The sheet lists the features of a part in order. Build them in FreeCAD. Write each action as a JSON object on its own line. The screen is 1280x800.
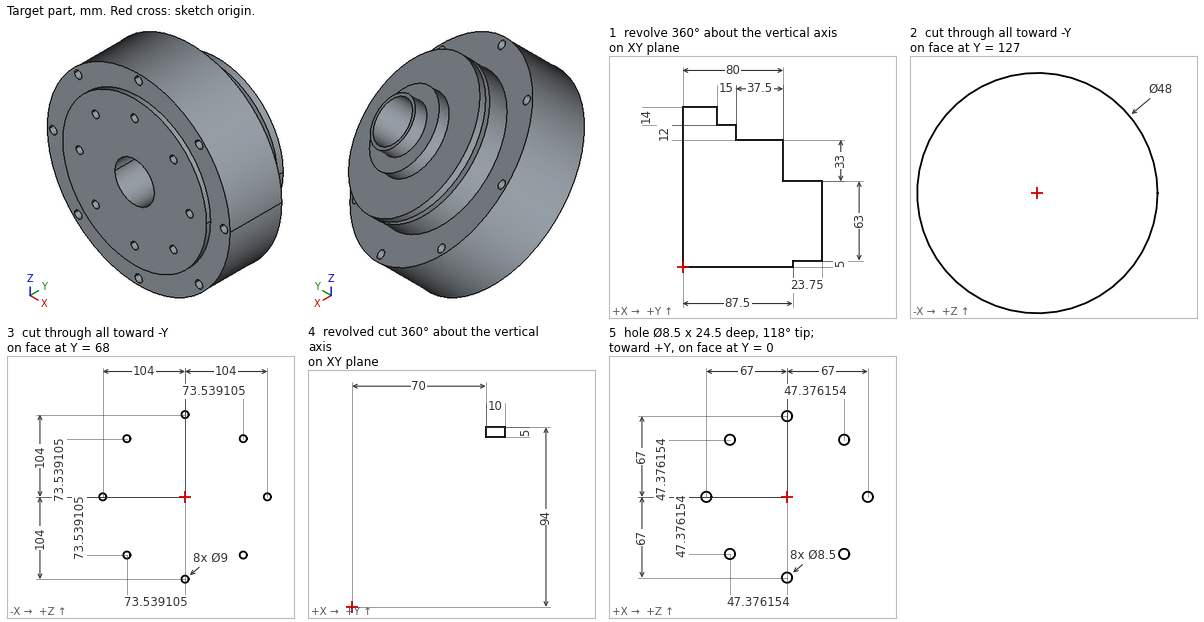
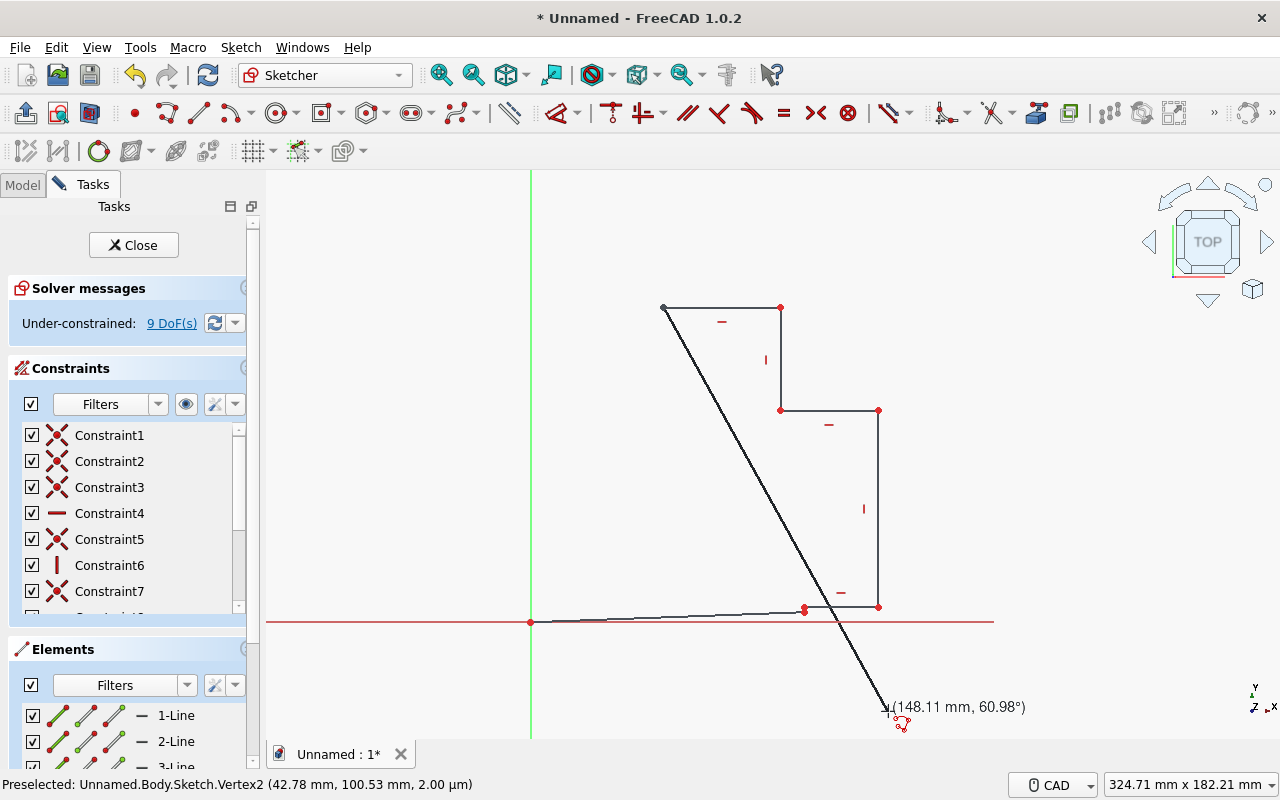
{"action": "left_click", "coordinate": [664, 269]}
{"action": "left_click", "coordinate": [617, 269]}
{"action": "left_click", "coordinate": [617, 226]}
{"action": "left_click", "coordinate": [540, 226]}
{"action": "left_click", "coordinate": [531, 622]}
{"action": "key", "text": "Escape"}
{"action": "key", "text": "Escape"}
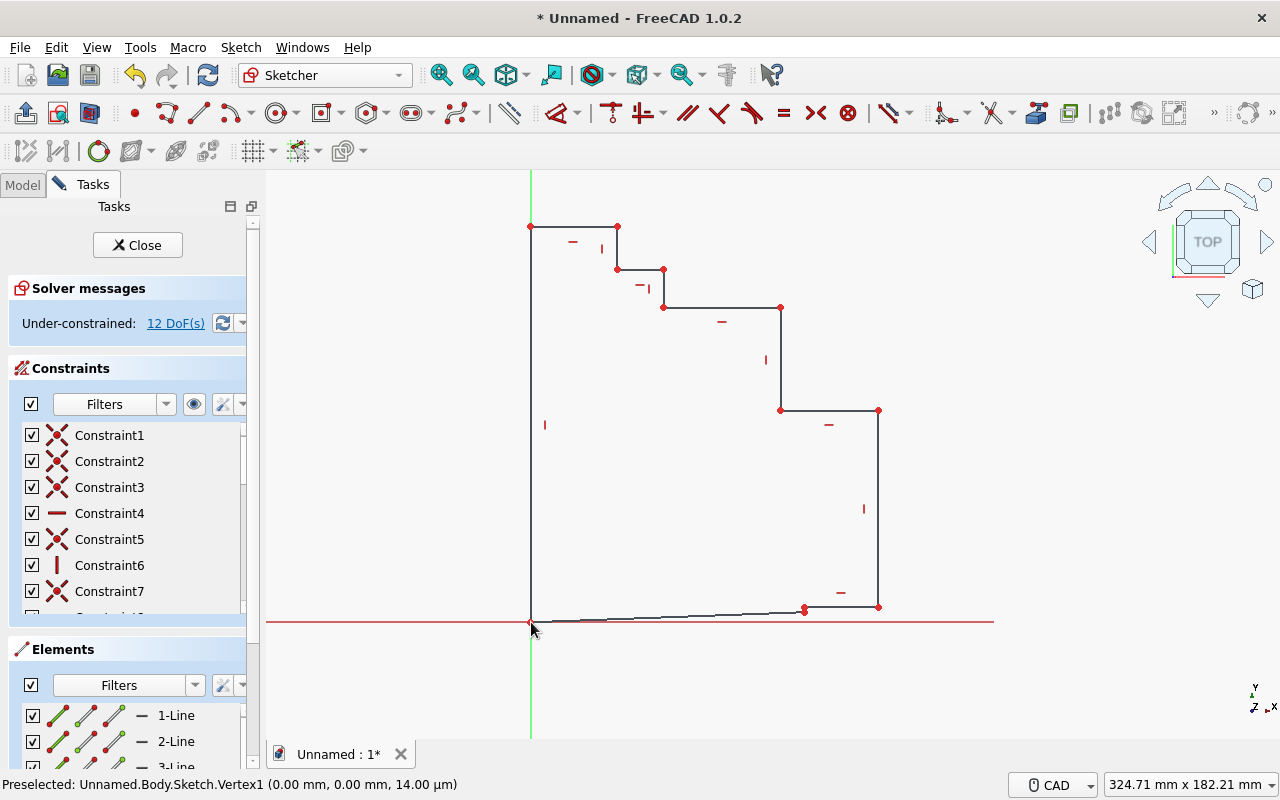
{"action": "left_click", "coordinate": [613, 619]}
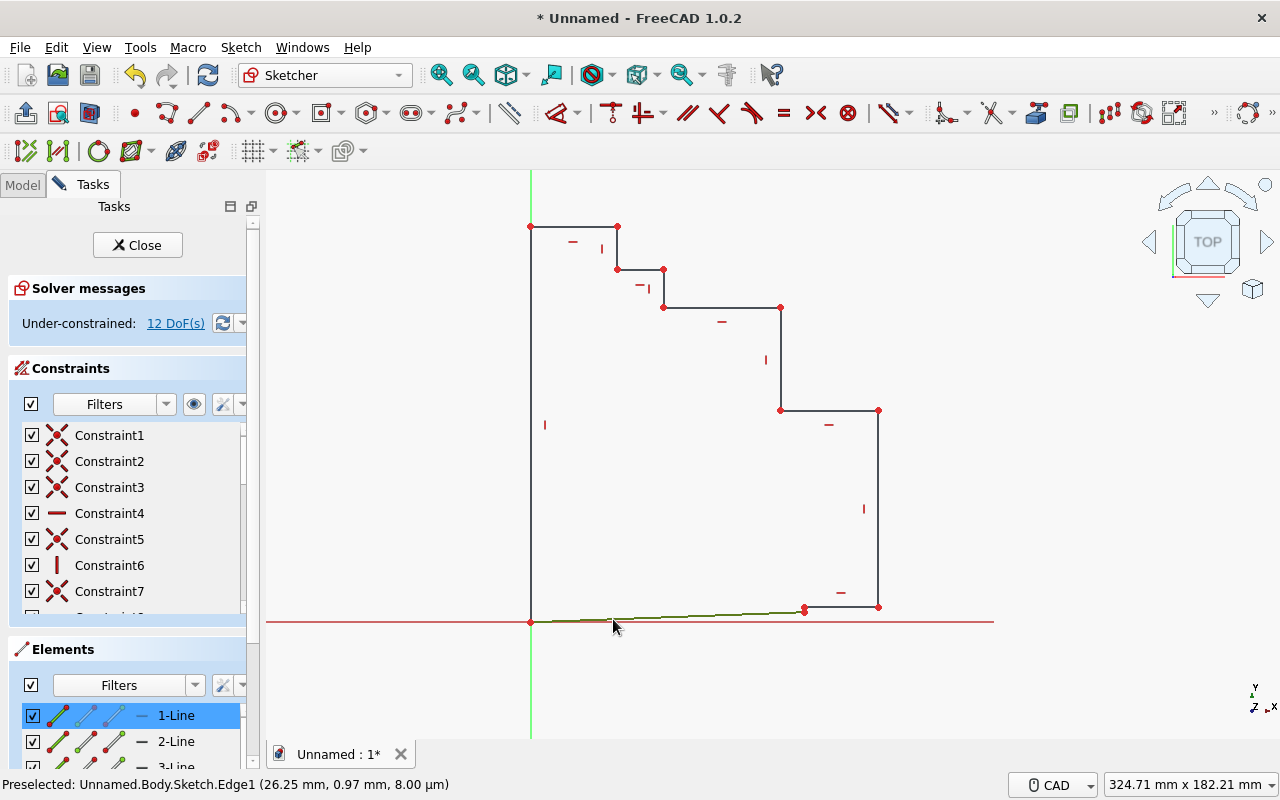
{"action": "key", "text": "h"}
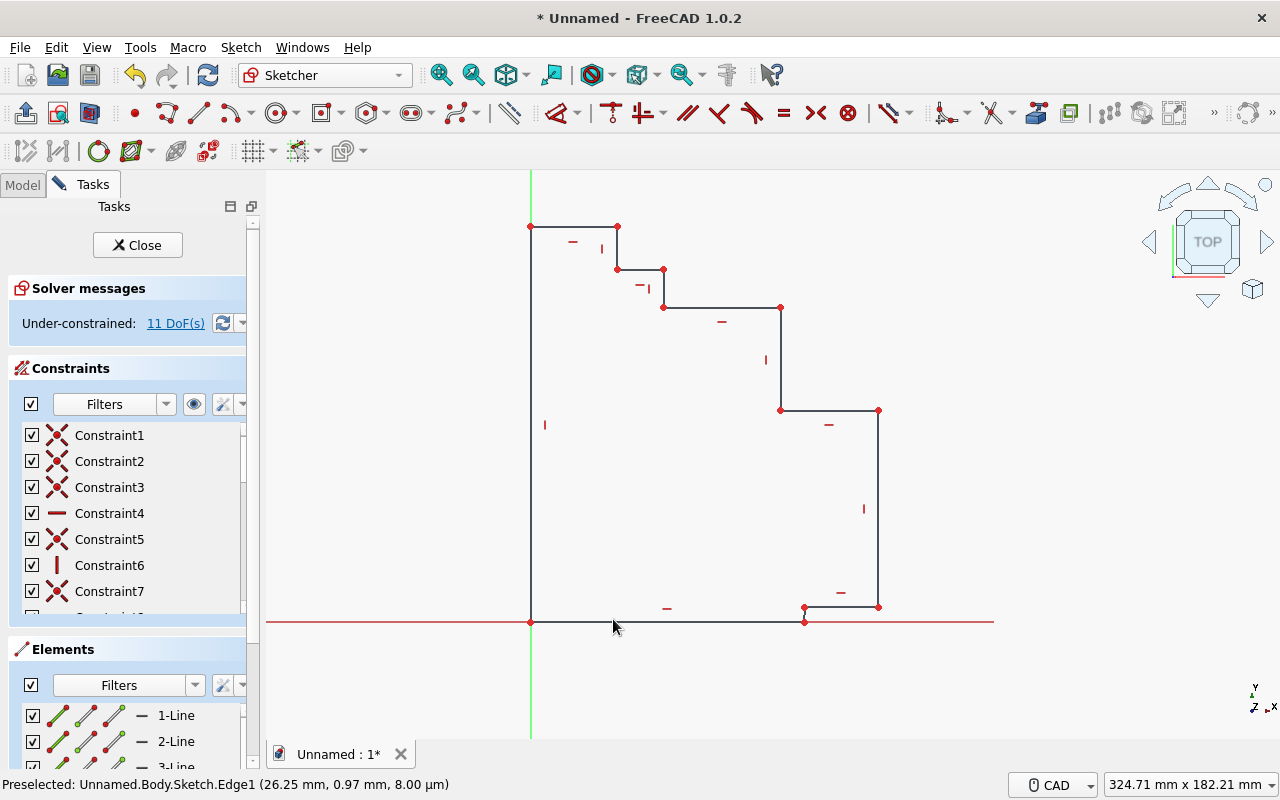
{"action": "scroll", "coordinate": [804, 615], "scroll_direction": "up", "scroll_amount": 4}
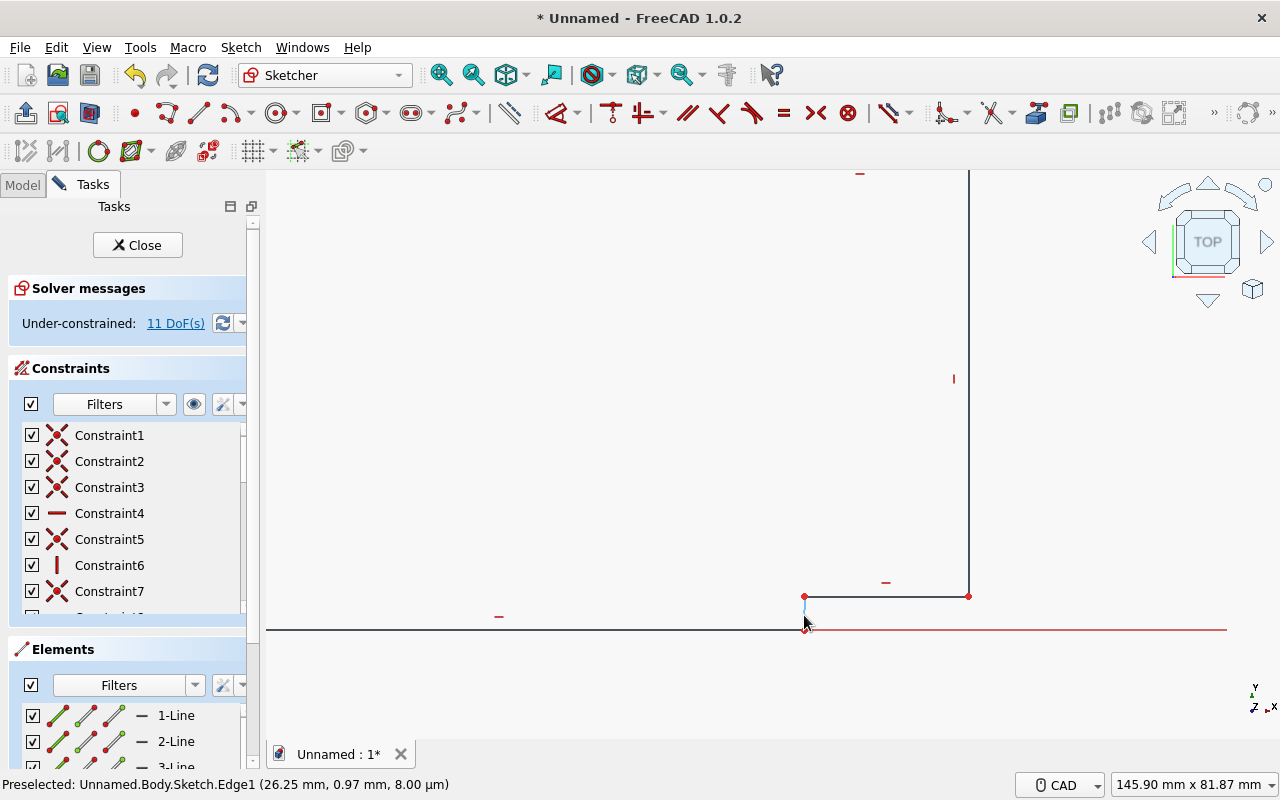
{"action": "left_click", "coordinate": [804, 613]}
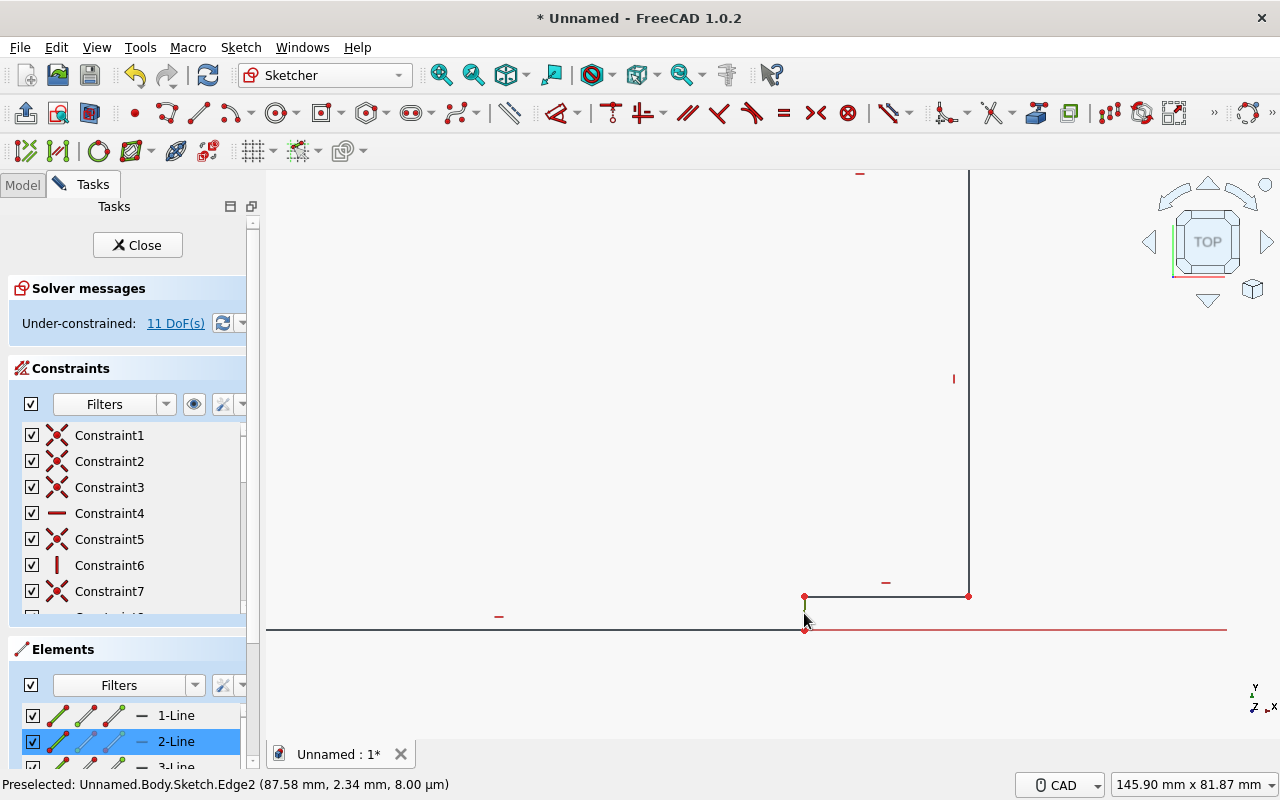
{"action": "left_click", "coordinate": [666, 114]}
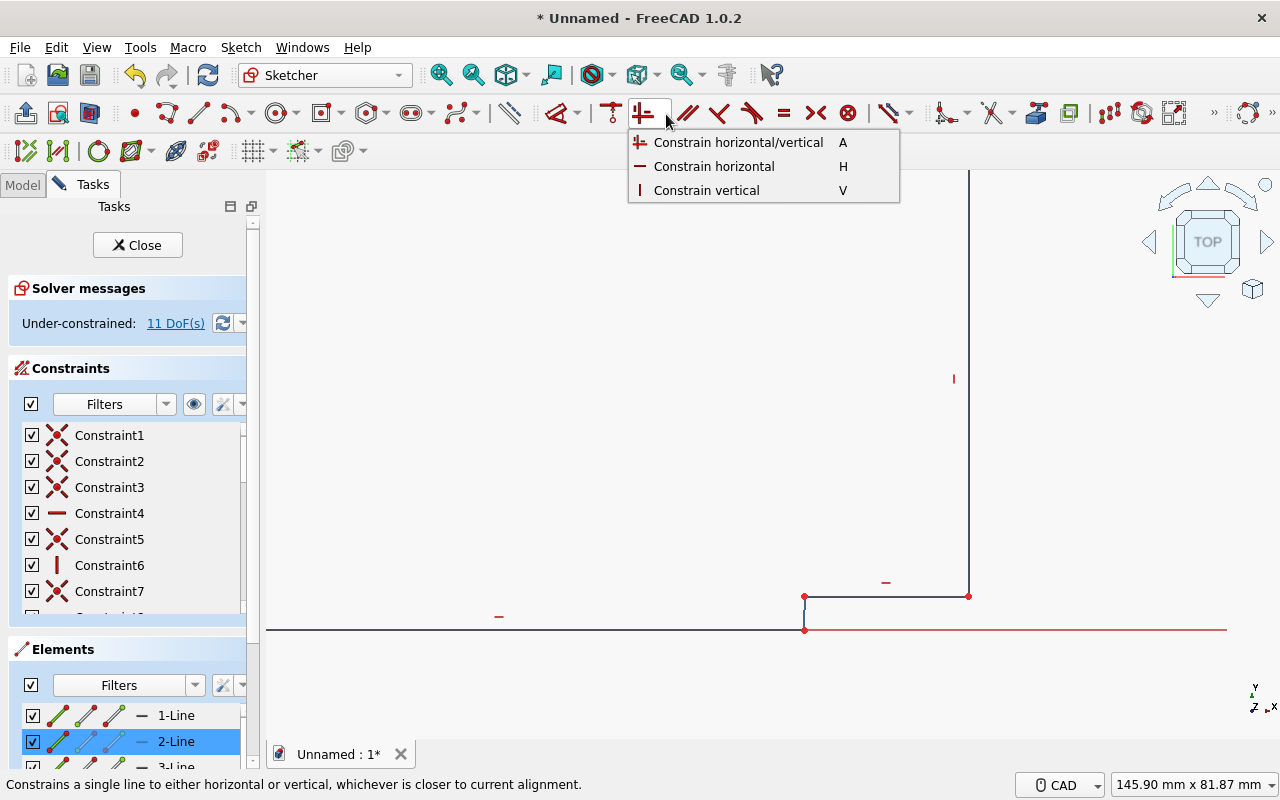
{"action": "left_click", "coordinate": [764, 190]}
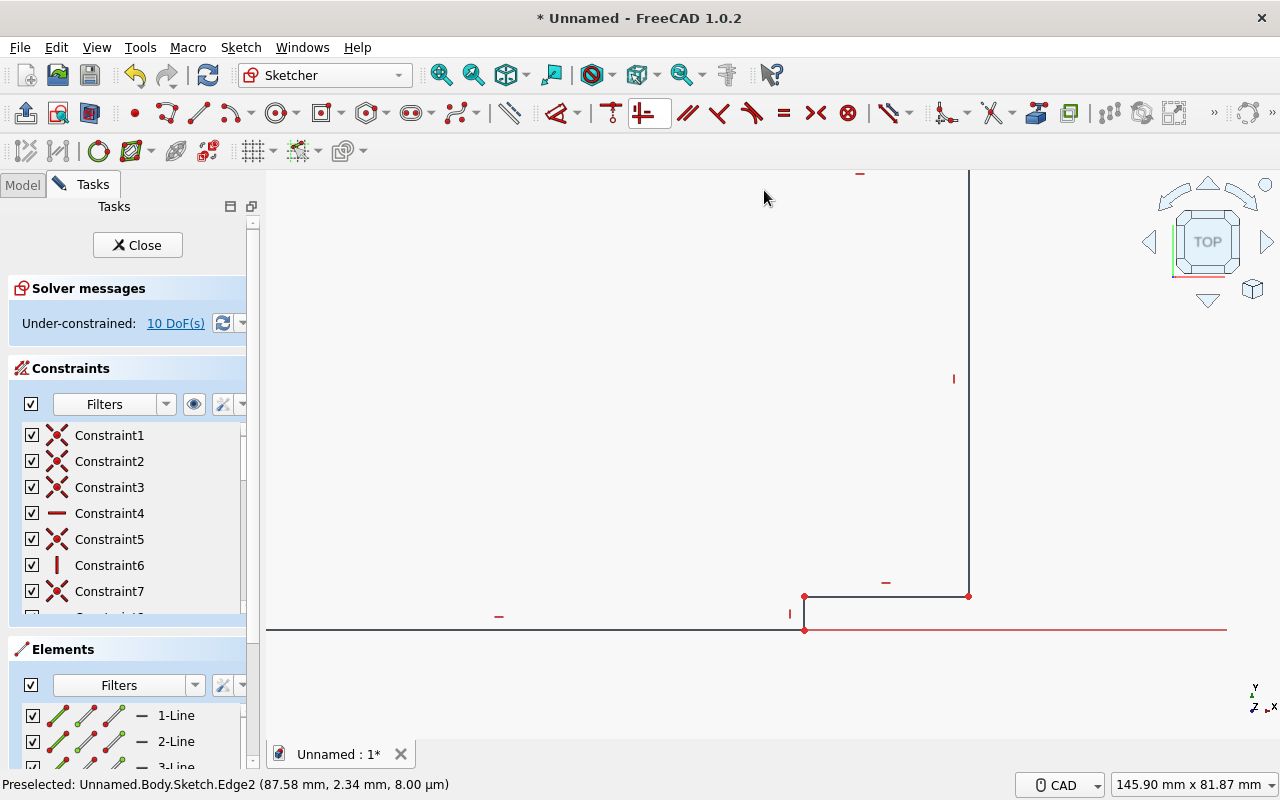
{"action": "left_click", "coordinate": [556, 114]}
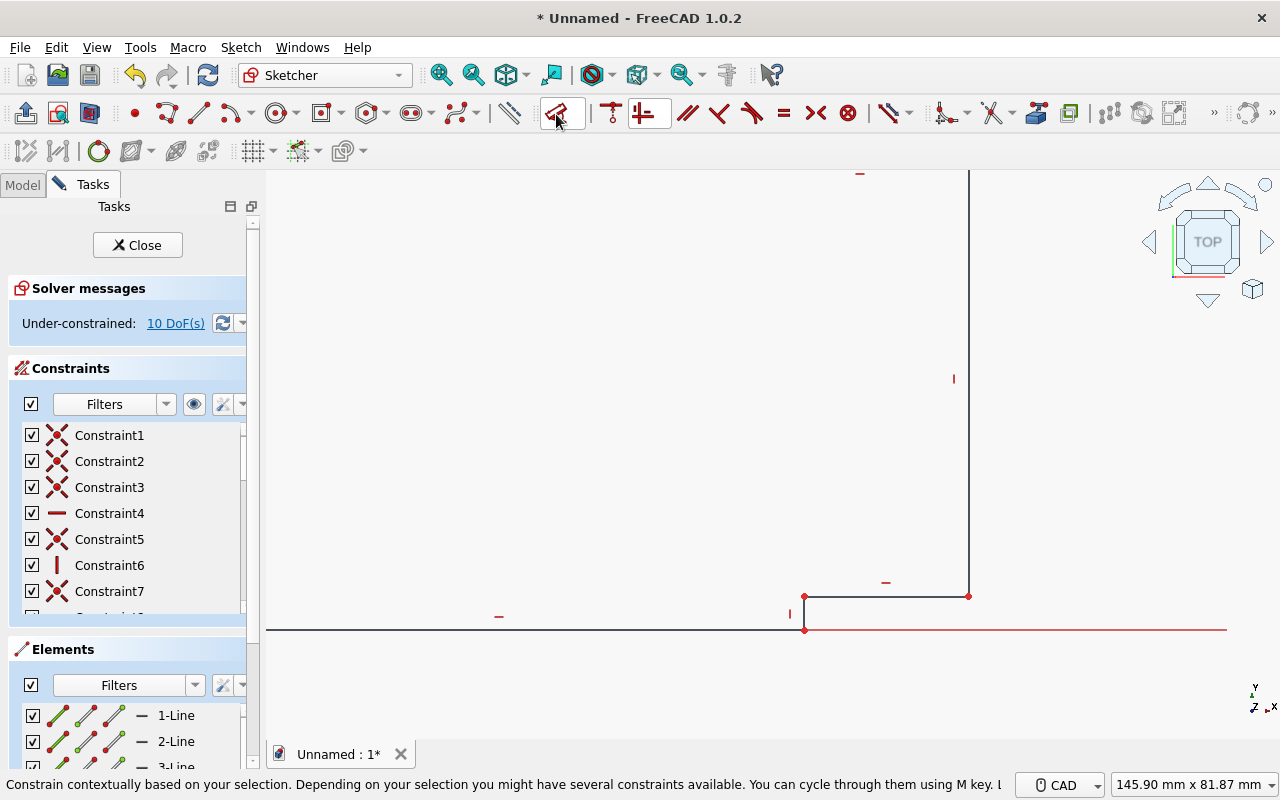
{"action": "scroll", "coordinate": [804, 620], "scroll_direction": "up", "scroll_amount": 2}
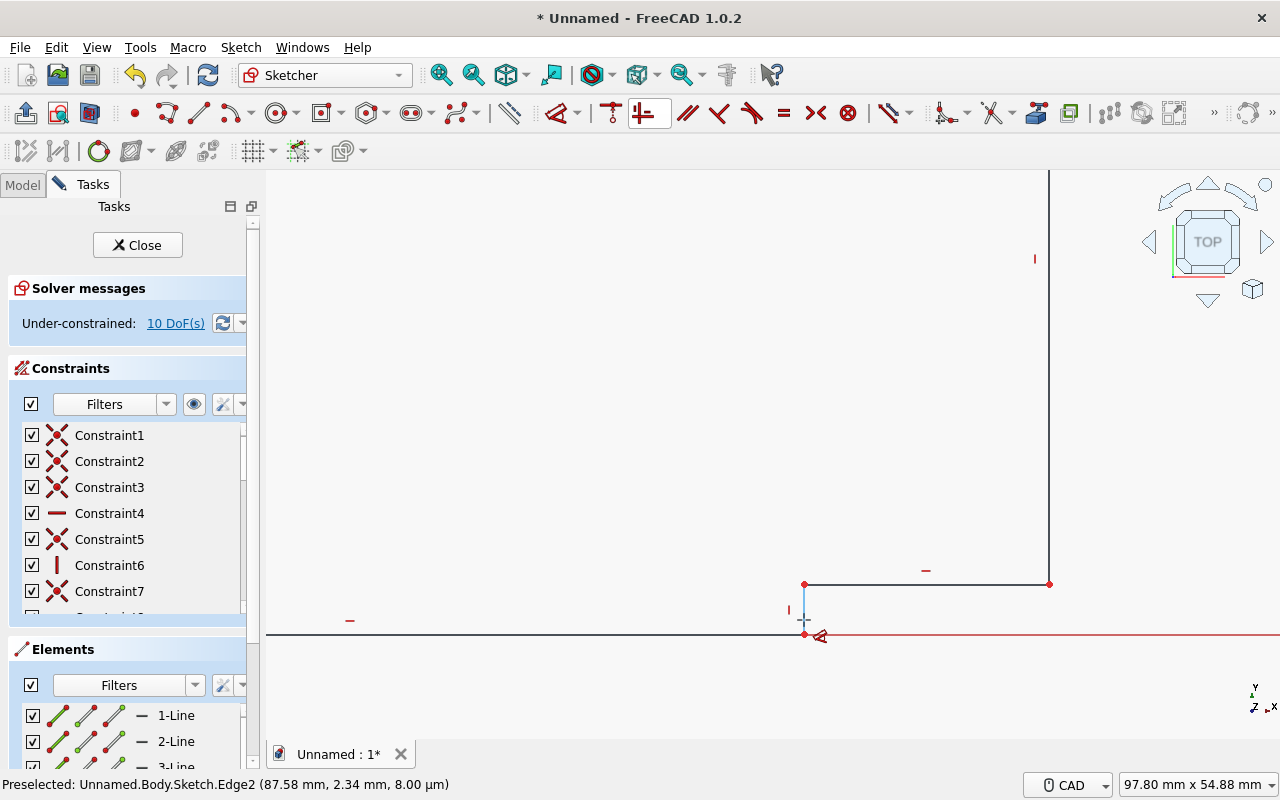
{"action": "left_click", "coordinate": [804, 620]}
{"action": "left_click", "coordinate": [838, 610]}